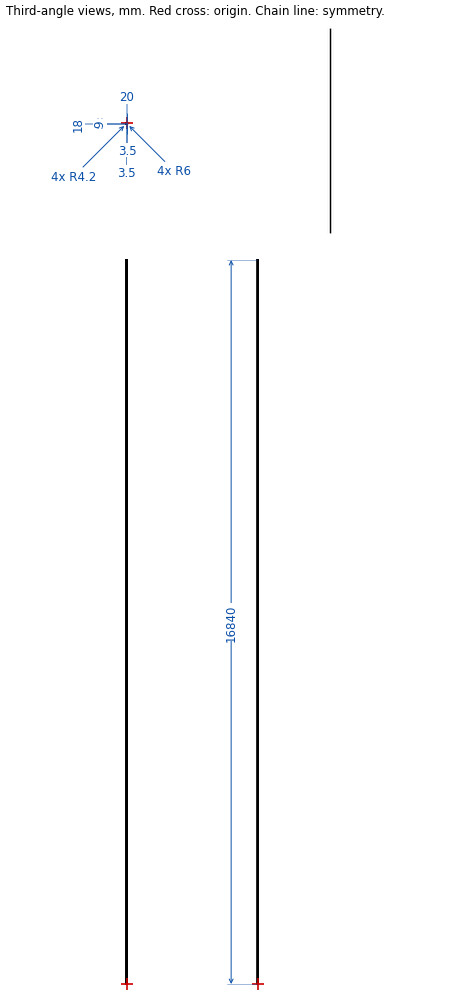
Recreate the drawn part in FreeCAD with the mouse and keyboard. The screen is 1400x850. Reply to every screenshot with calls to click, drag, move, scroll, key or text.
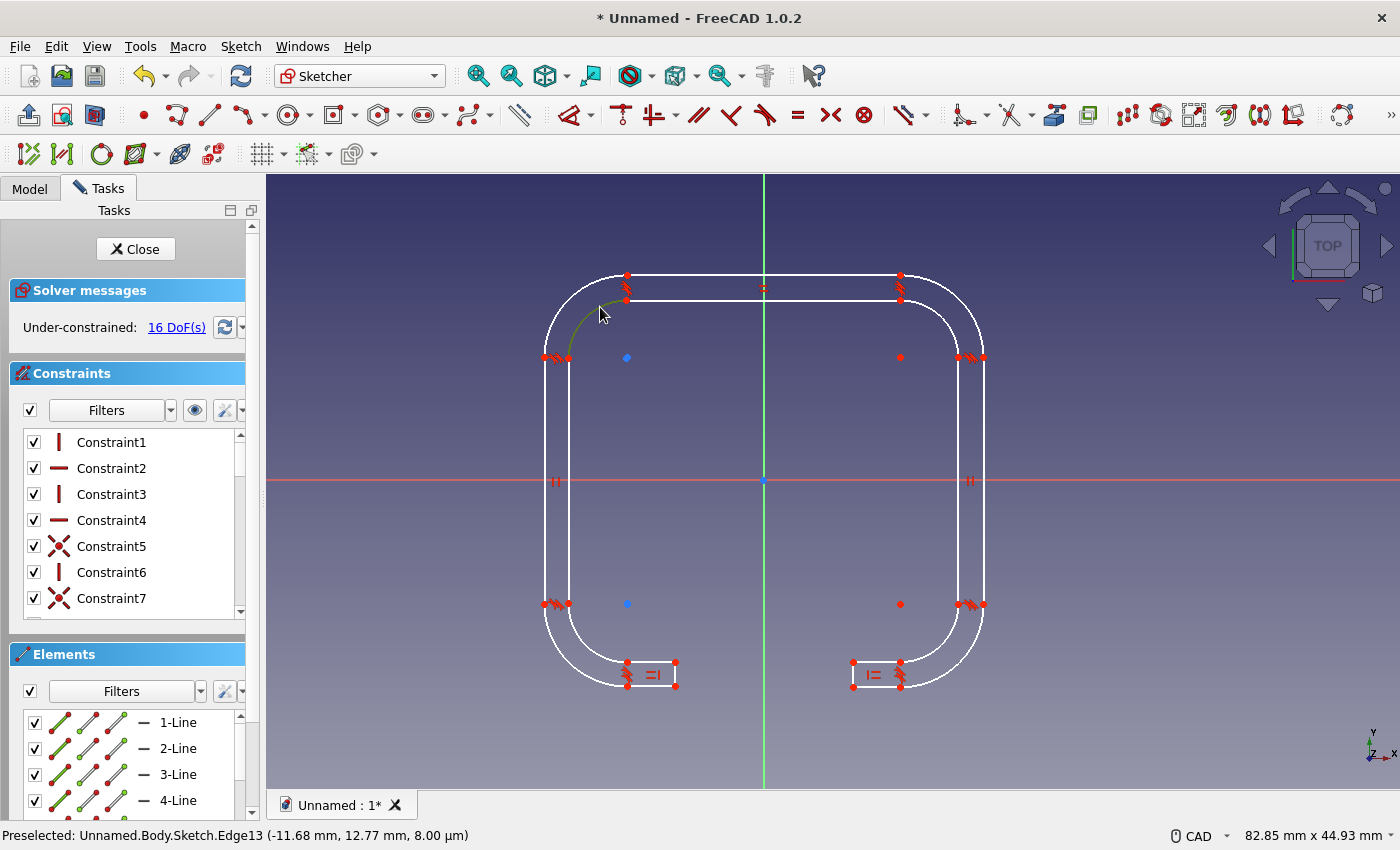
click(590, 284)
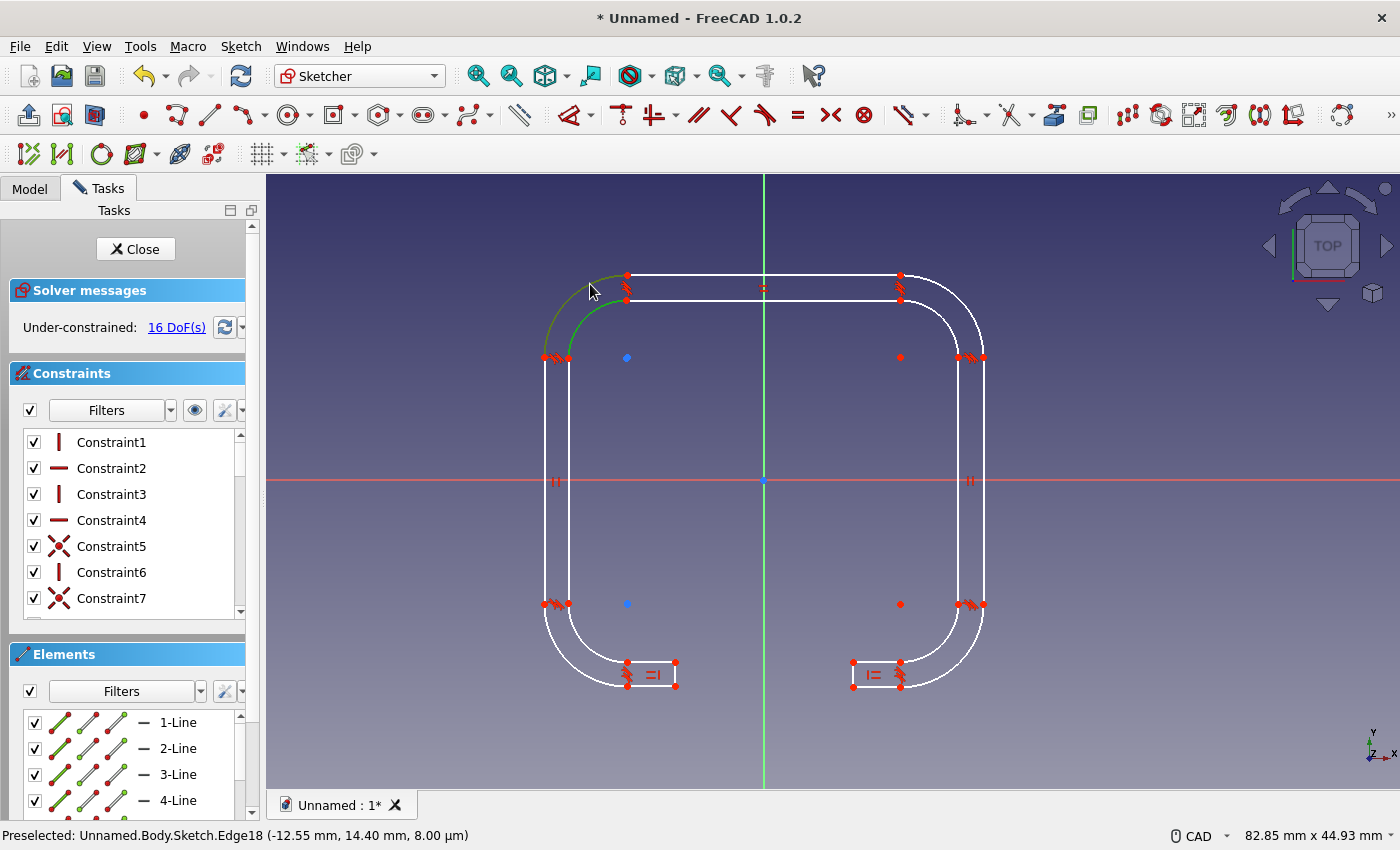
click(621, 116)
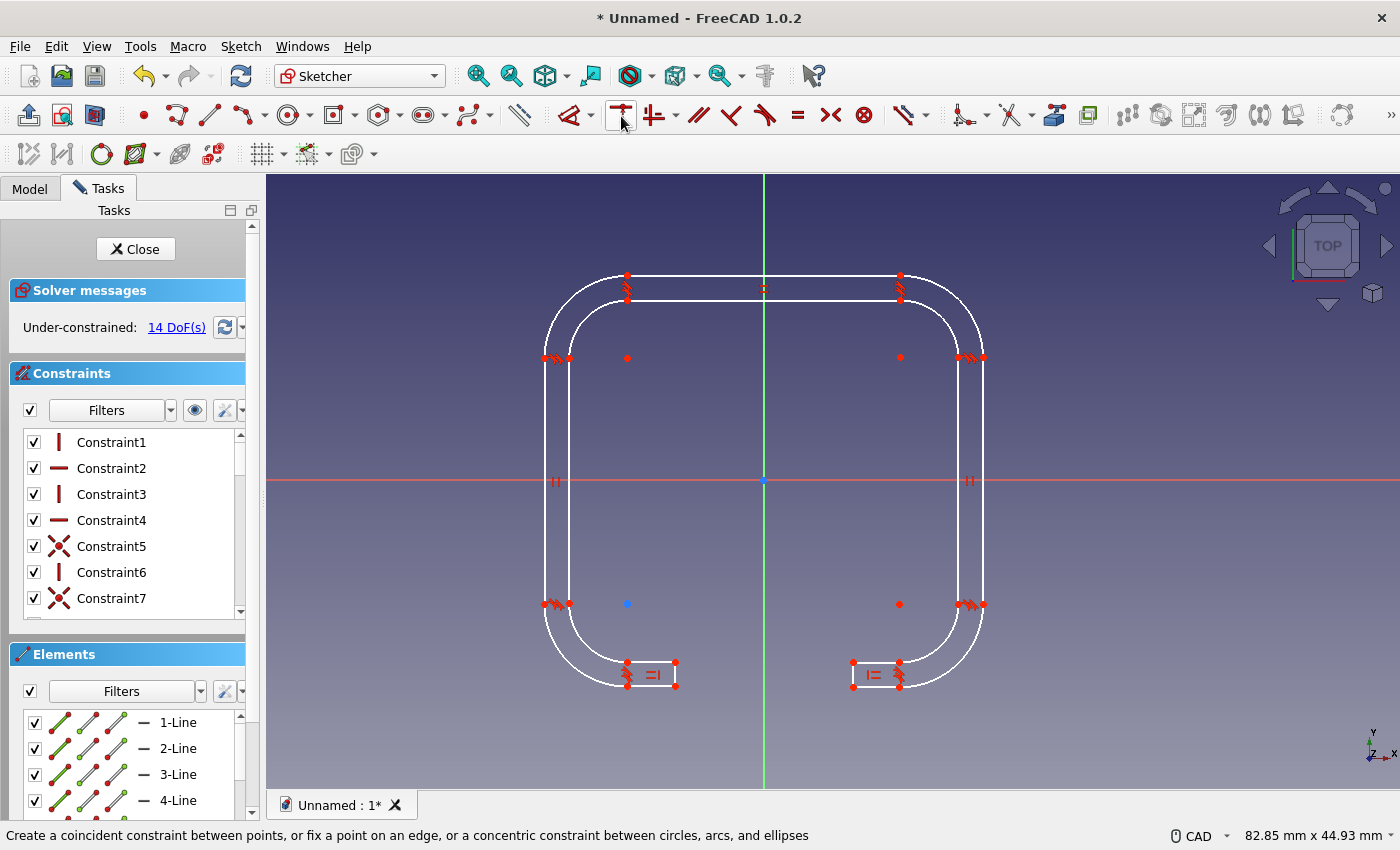
click(554, 641)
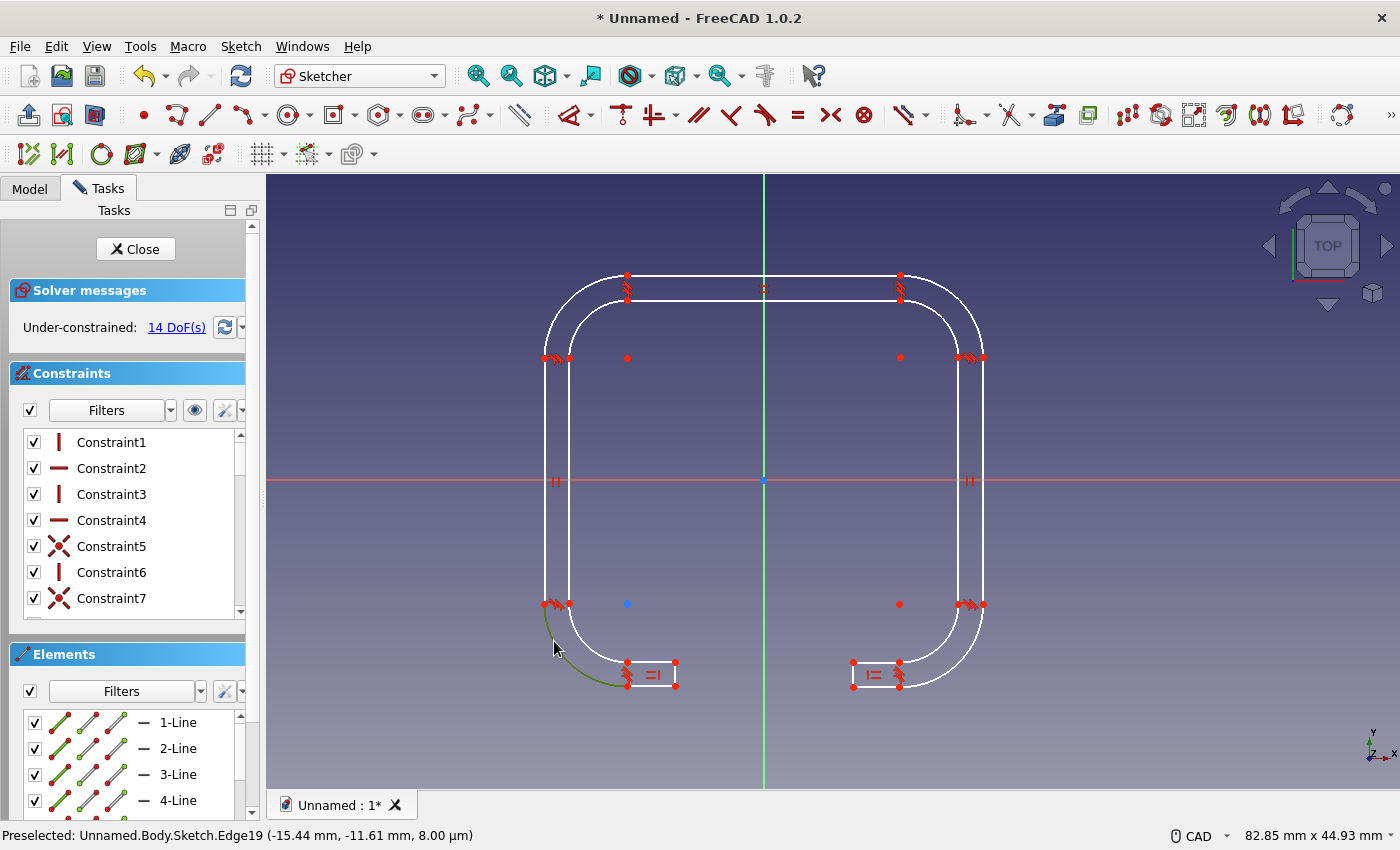
click(576, 630)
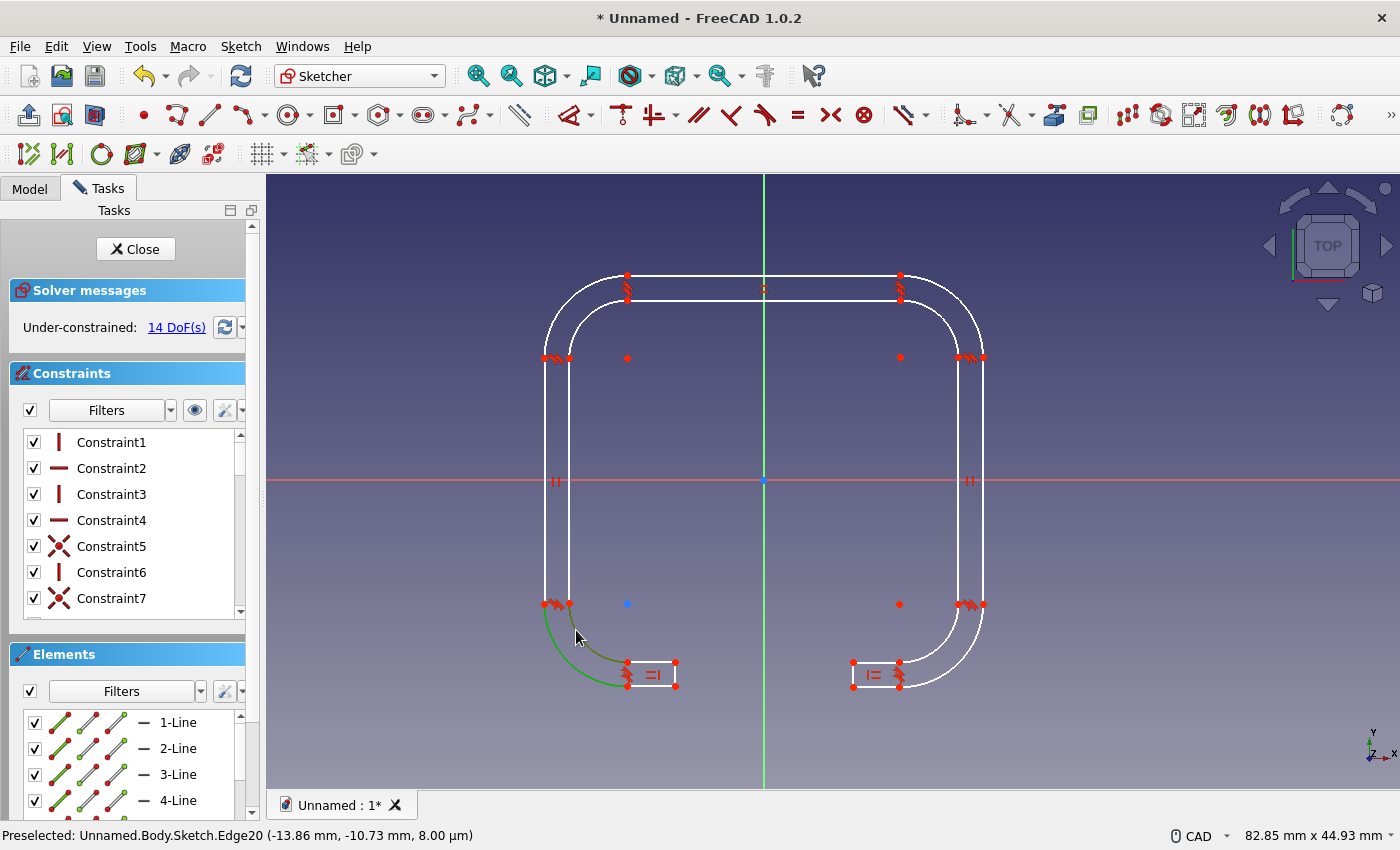
click(621, 116)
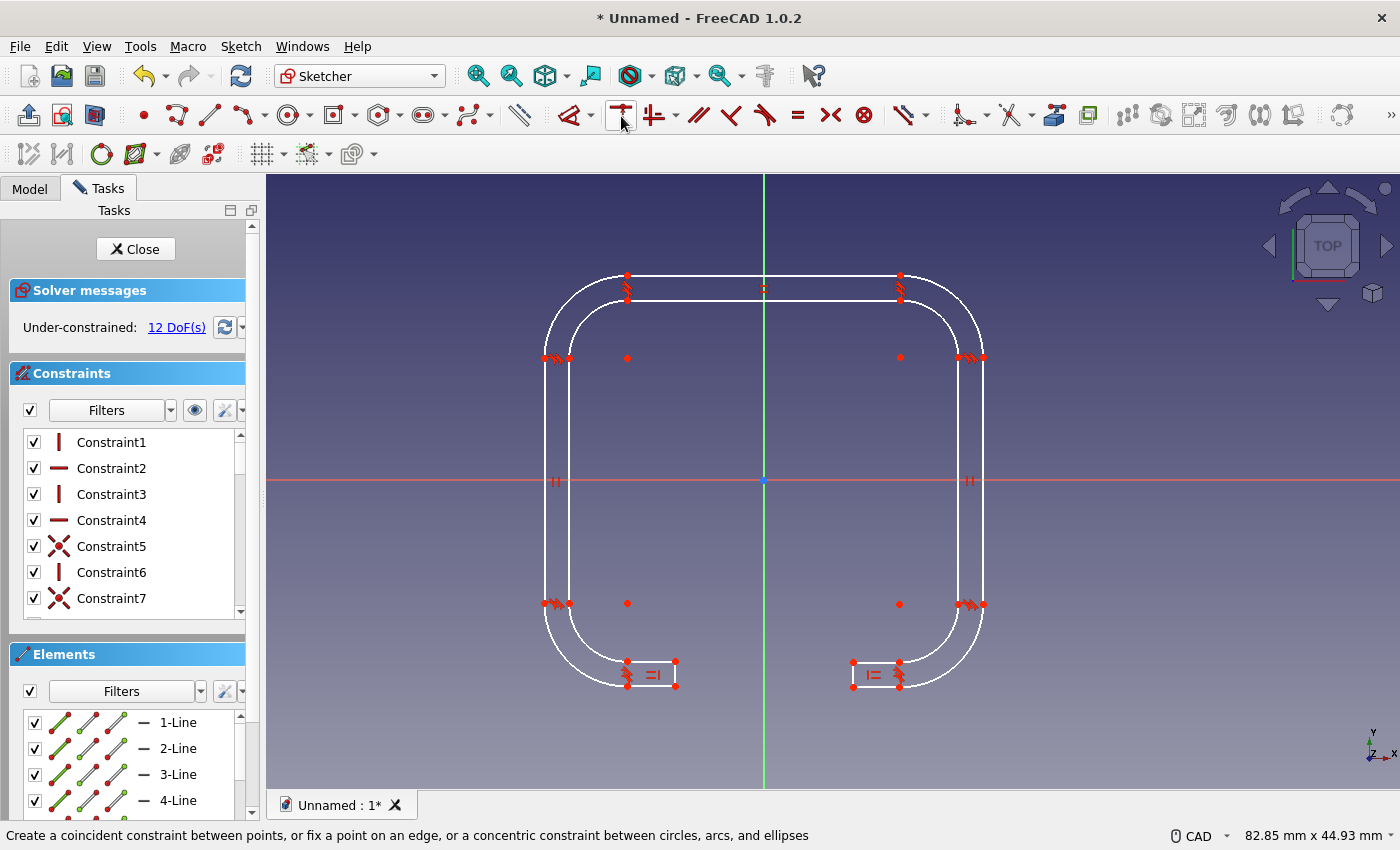
click(601, 307)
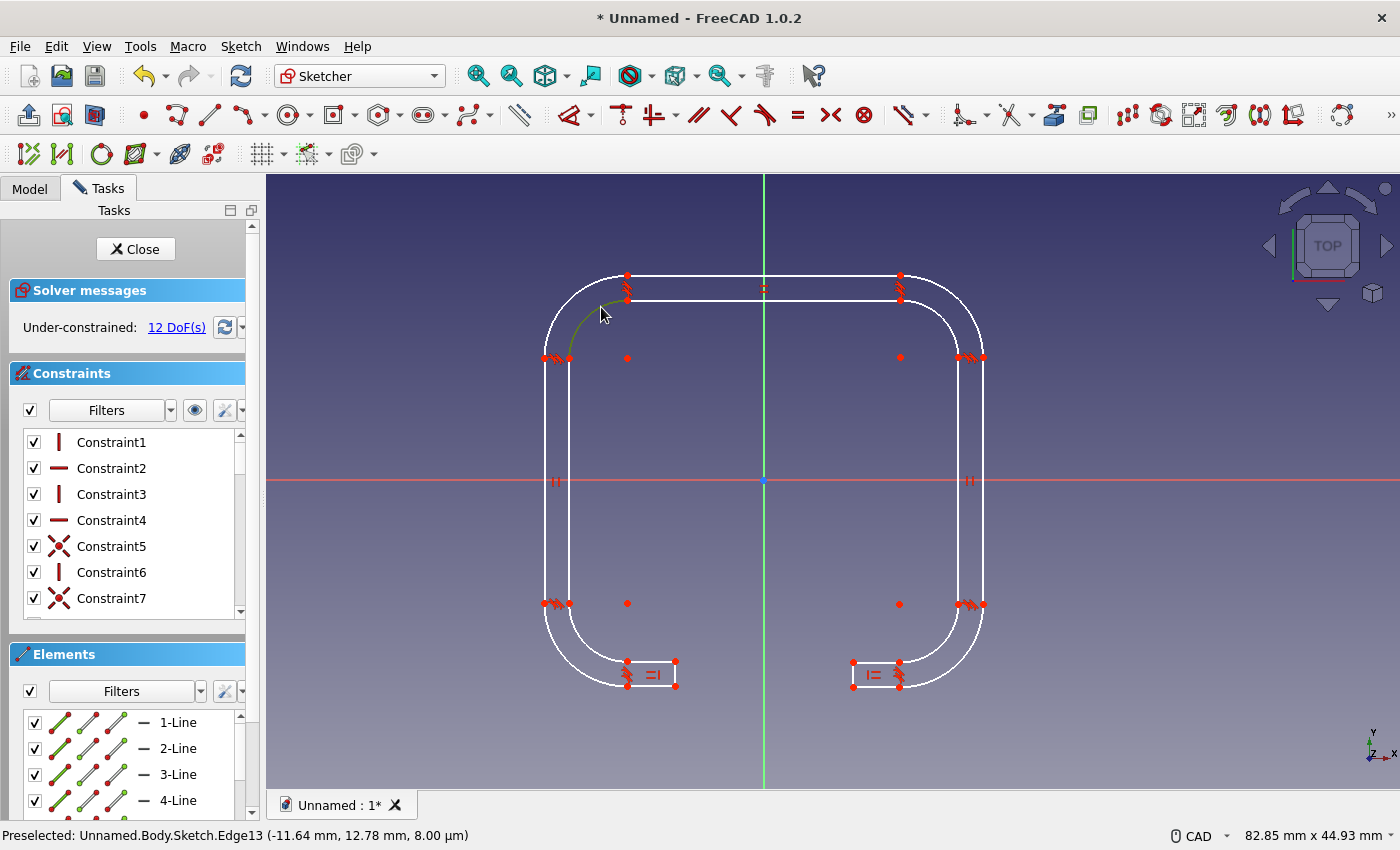
click(952, 332)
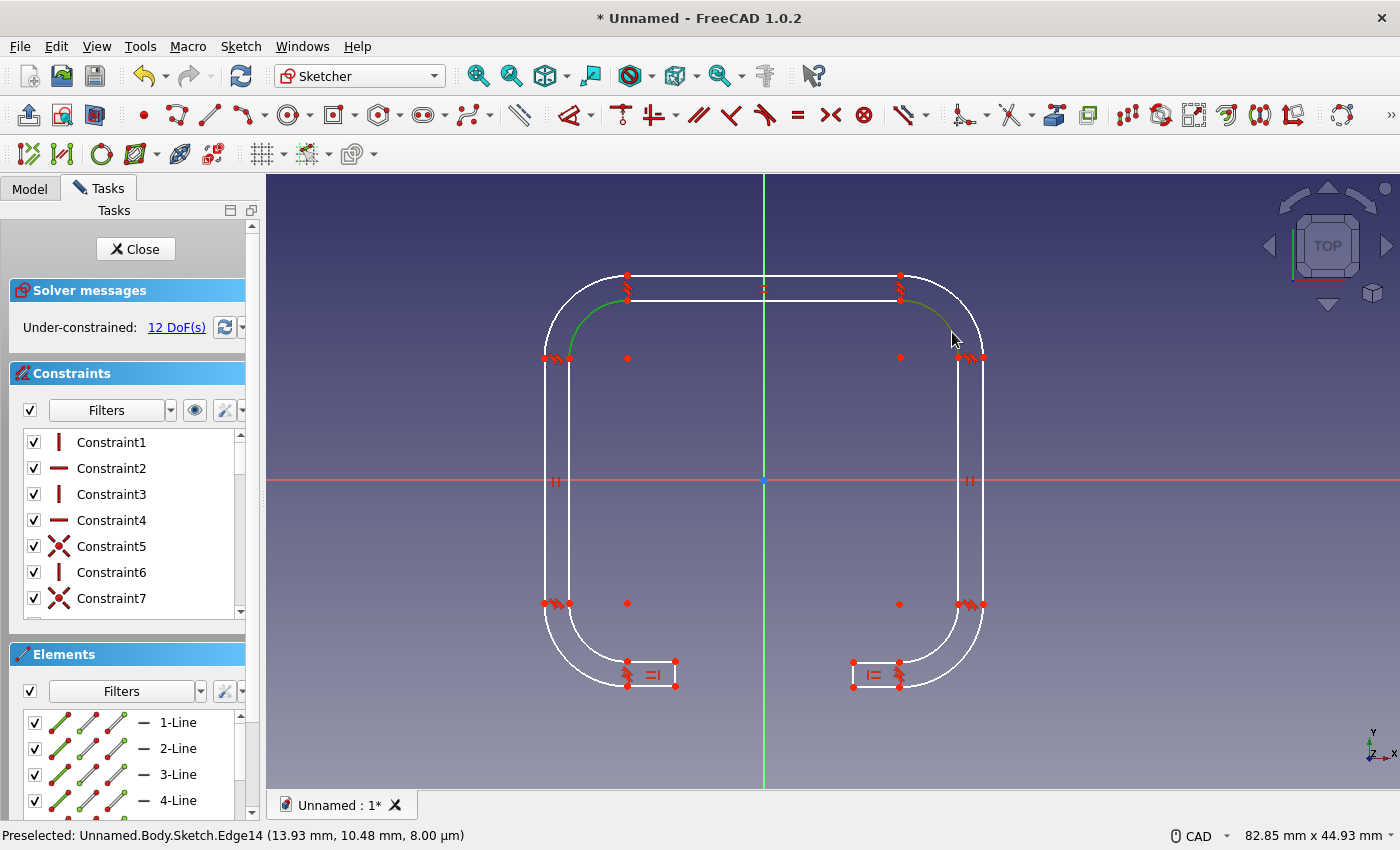
click(926, 656)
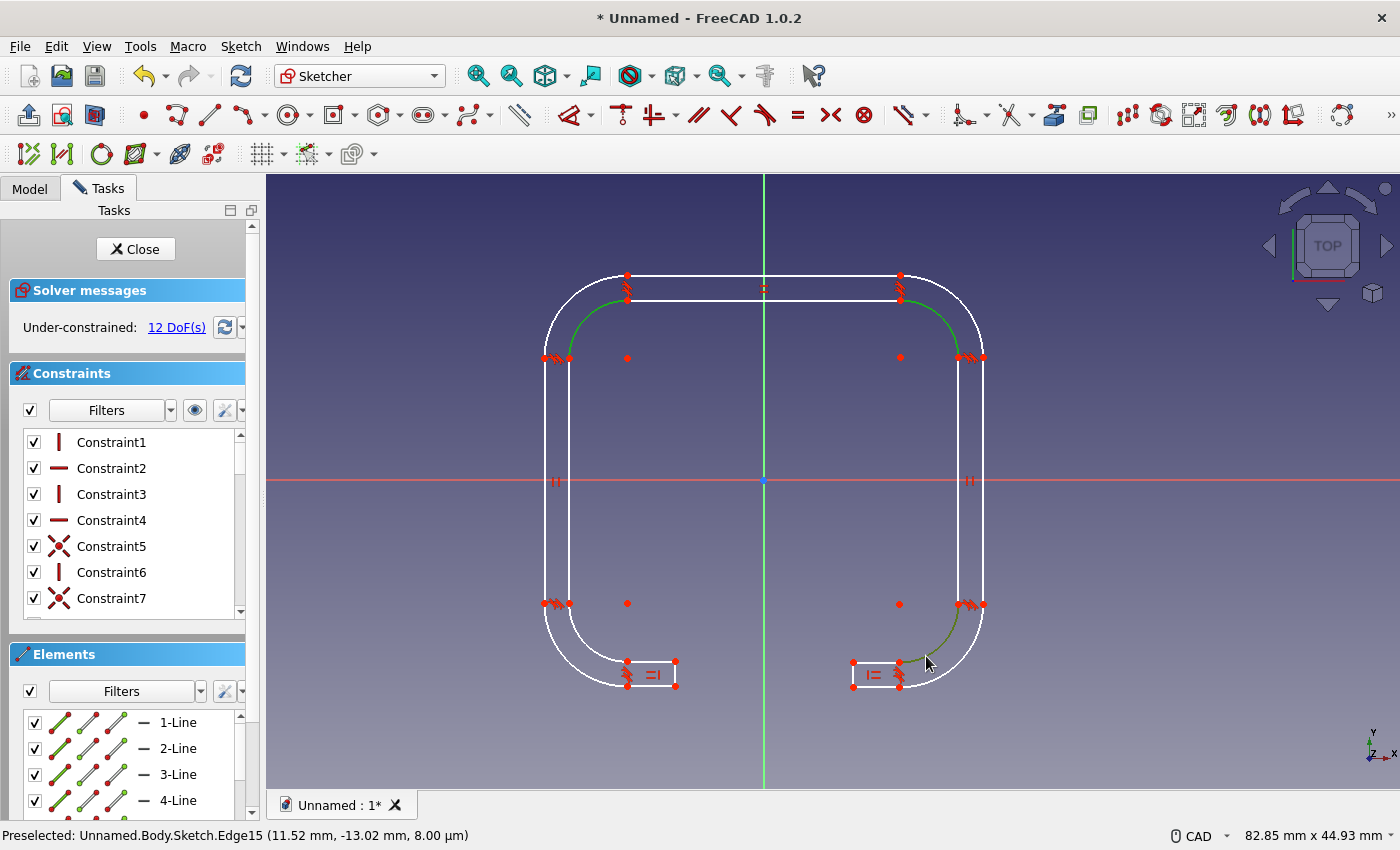
click(576, 630)